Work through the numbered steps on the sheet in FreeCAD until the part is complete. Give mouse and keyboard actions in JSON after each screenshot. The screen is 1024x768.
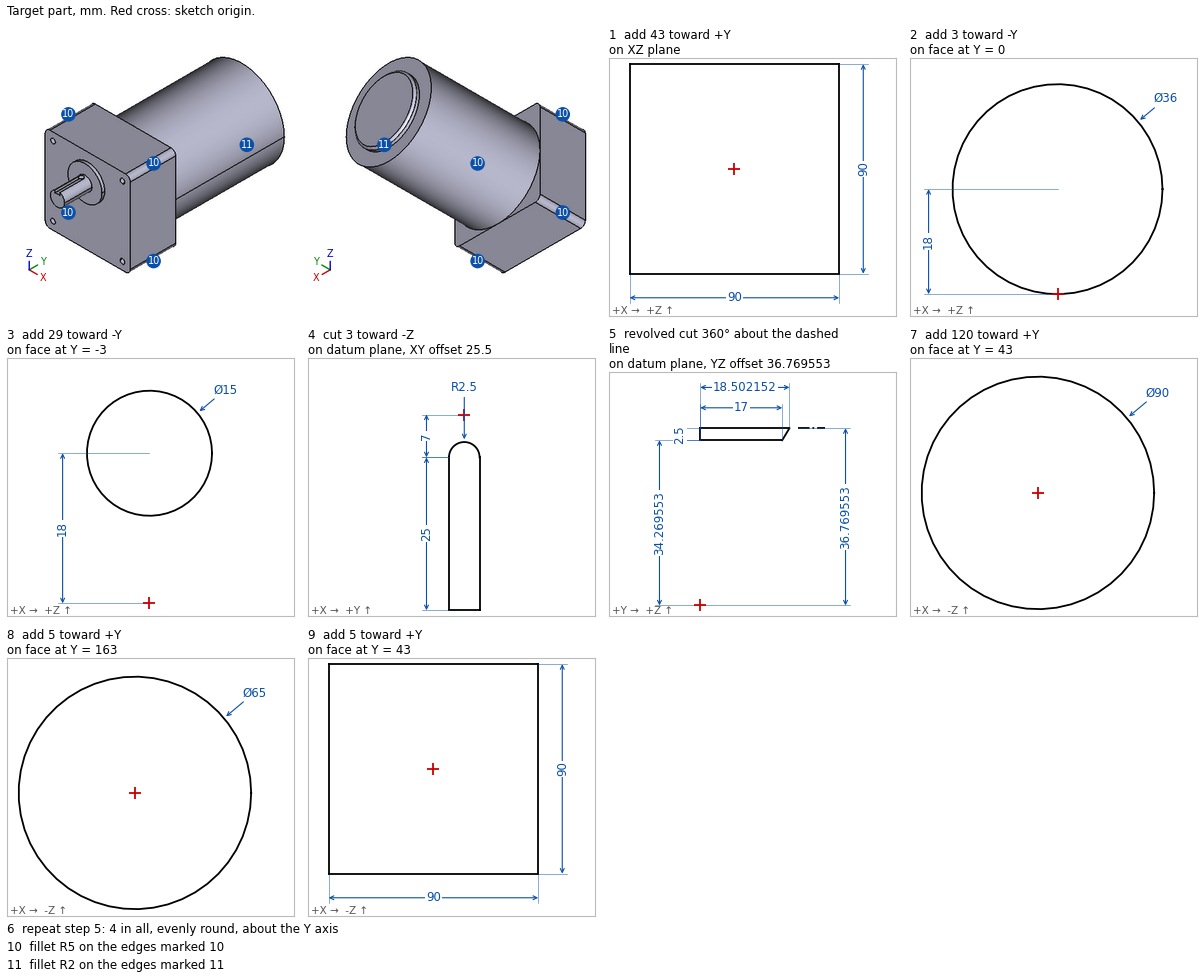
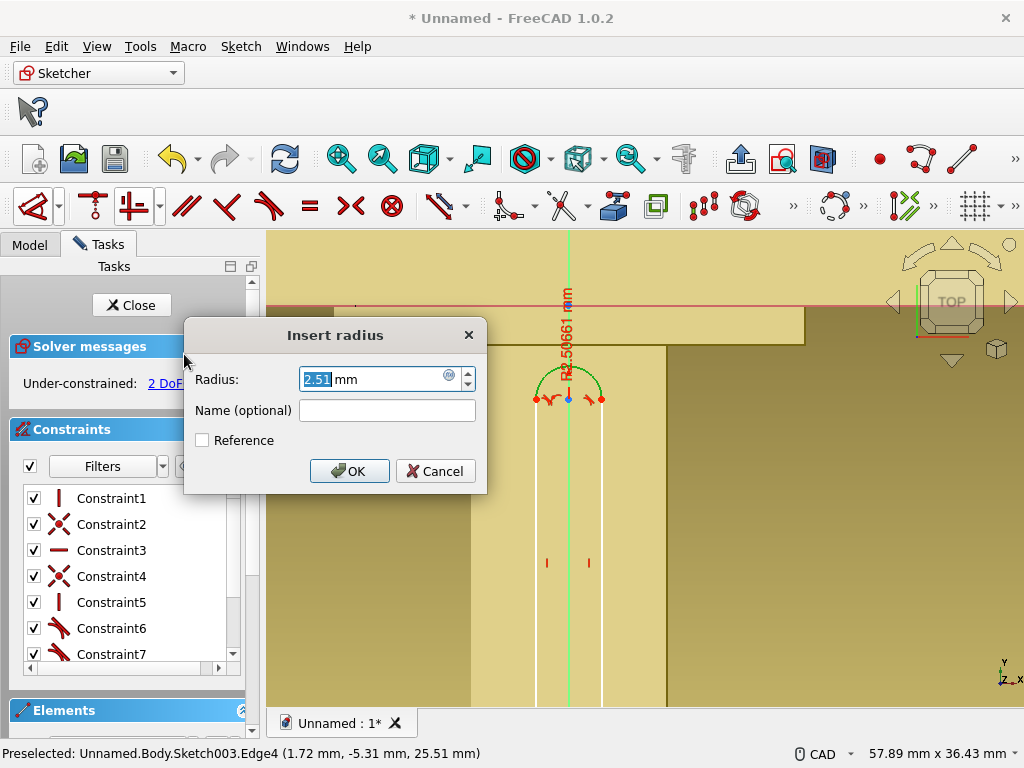
{"action": "type", "text": "2.5"}
{"action": "key", "text": "Return"}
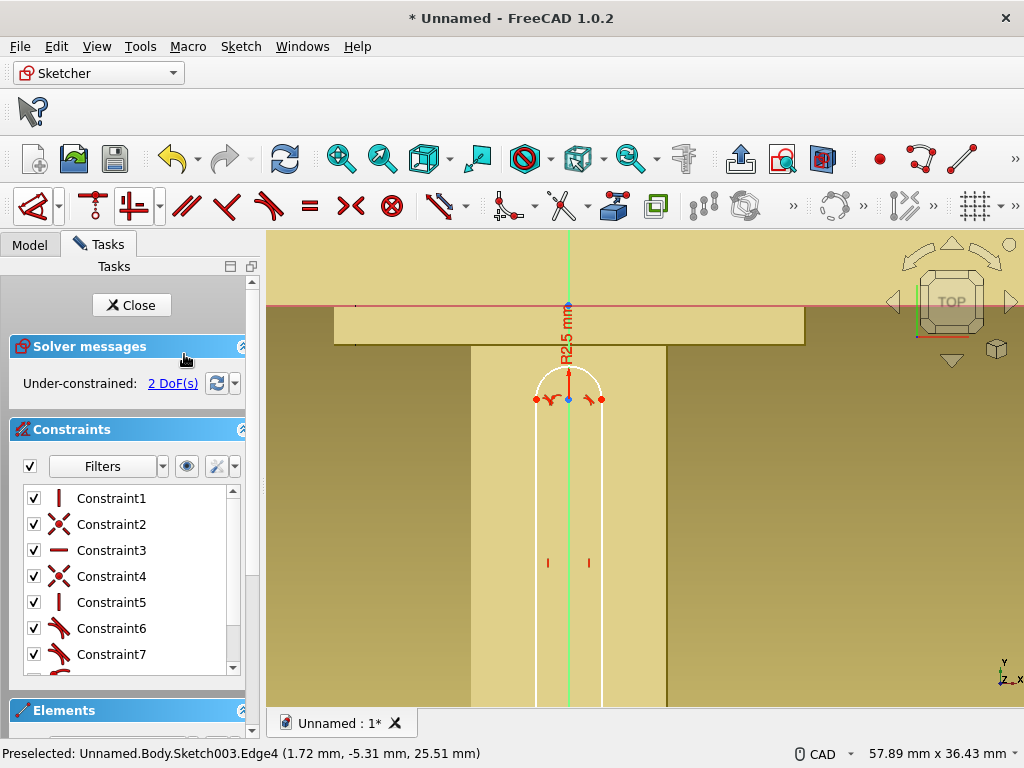
{"action": "left_click", "coordinate": [536, 497]}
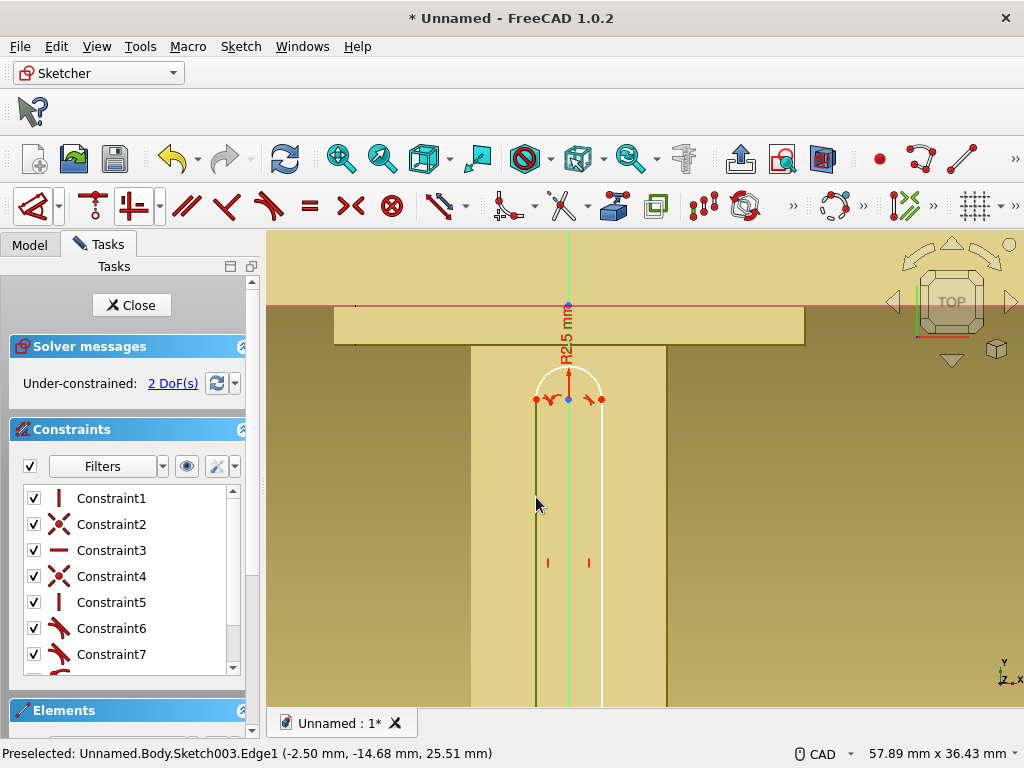
{"action": "left_click", "coordinate": [58, 206]}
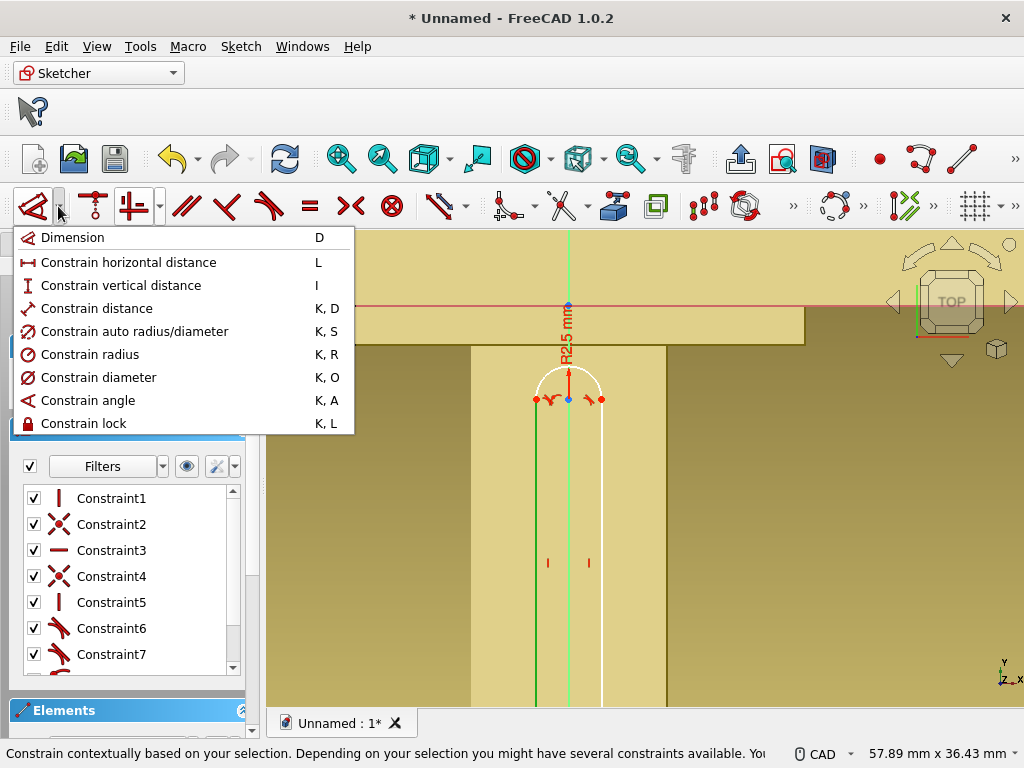
{"action": "left_click", "coordinate": [184, 286]}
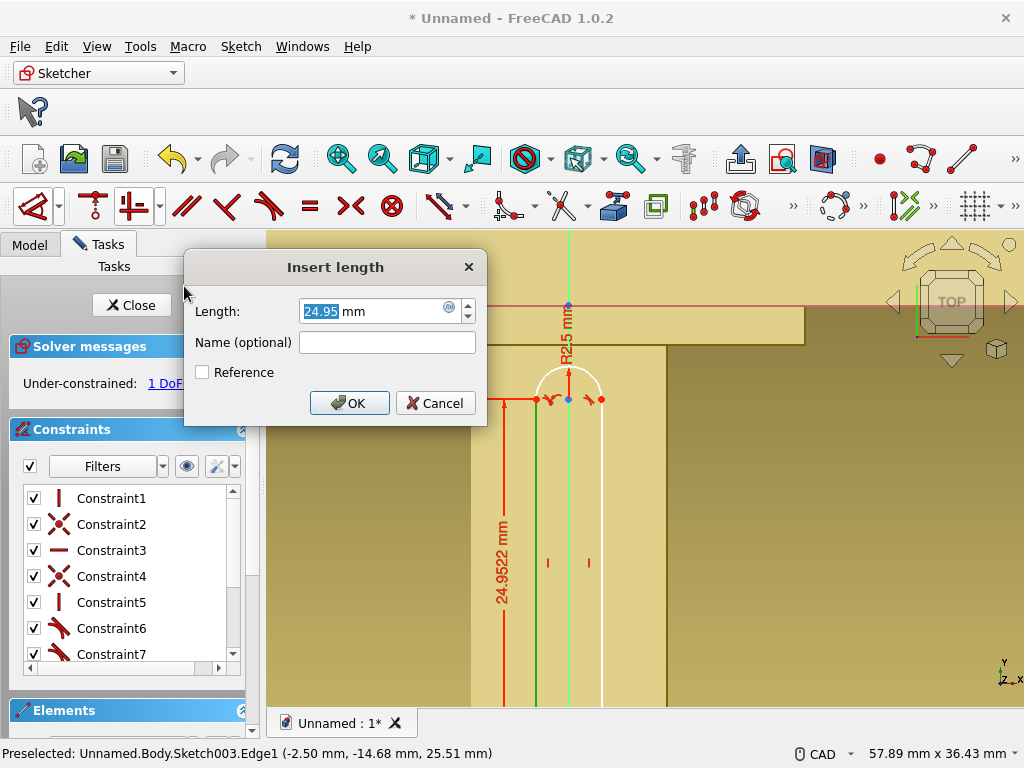
{"action": "type", "text": "25"}
{"action": "key", "text": "Return"}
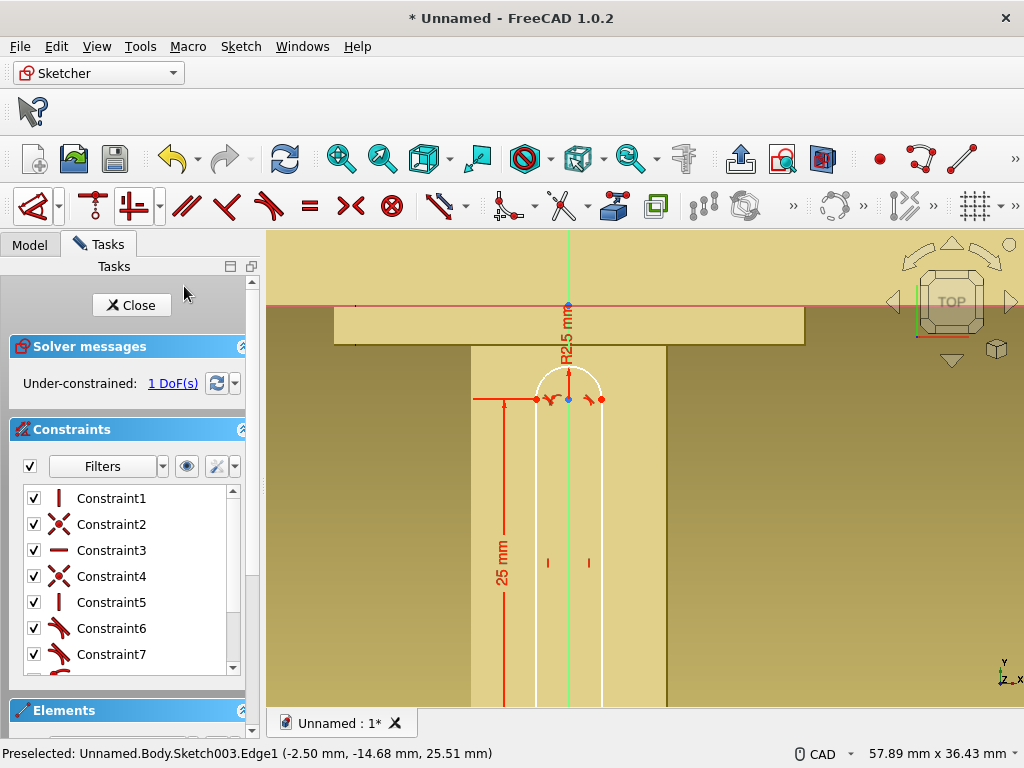
{"action": "left_click", "coordinate": [536, 399]}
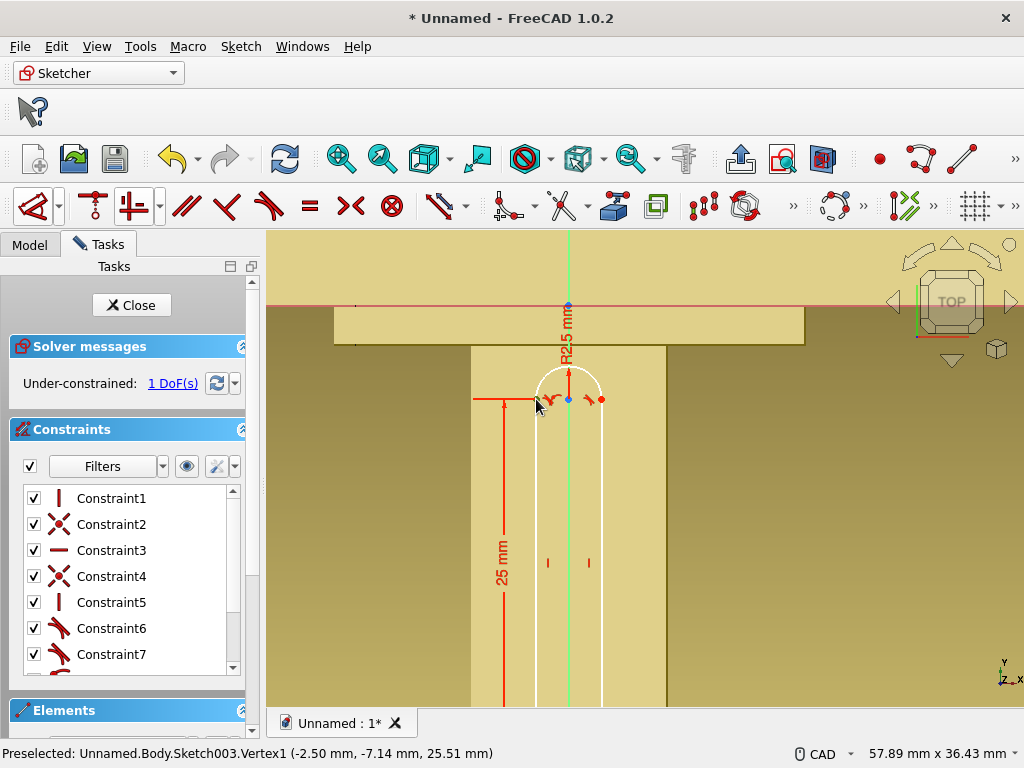
{"action": "left_click", "coordinate": [58, 206]}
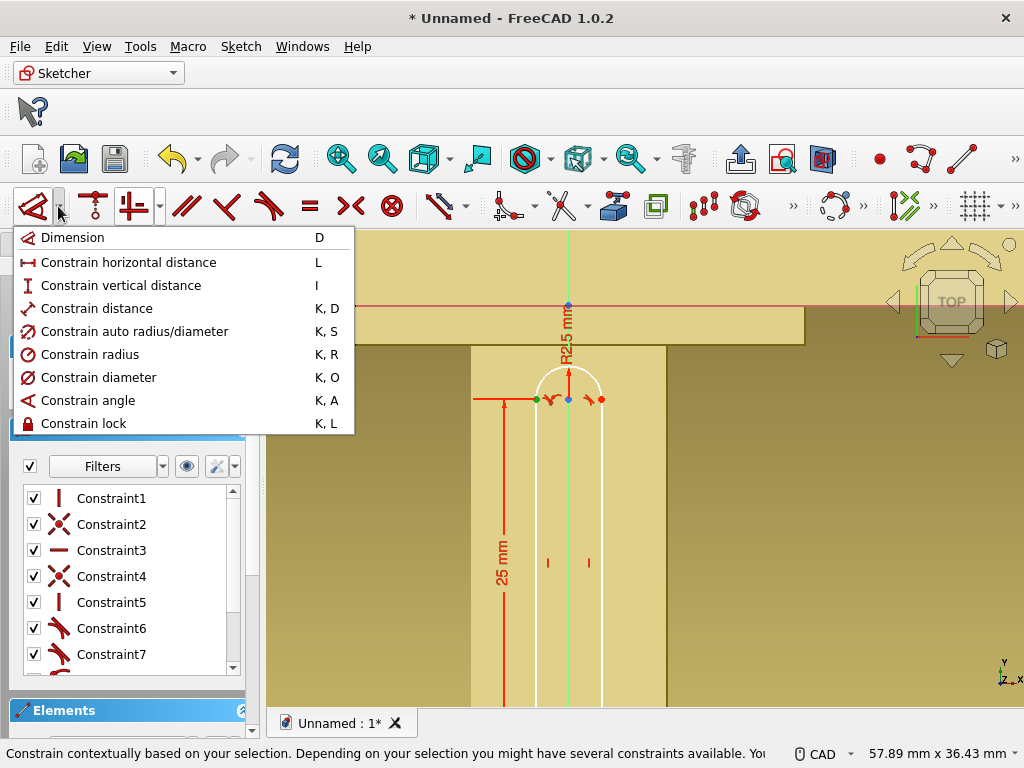
{"action": "left_click", "coordinate": [184, 286]}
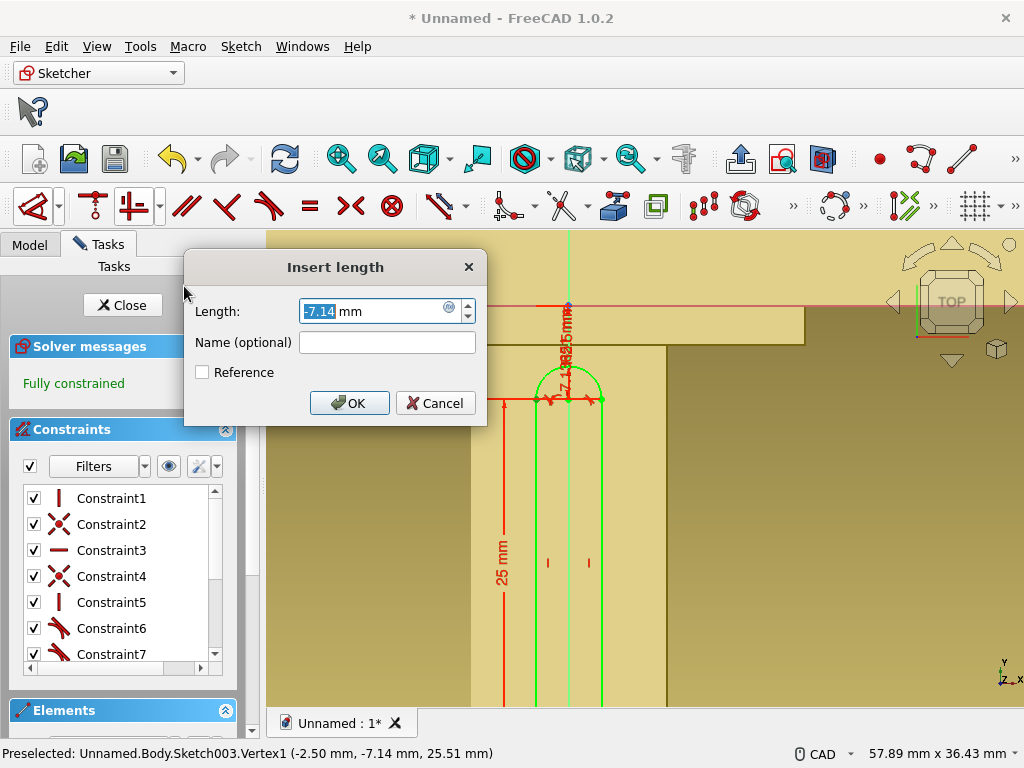
{"action": "type", "text": "-7"}
{"action": "key", "text": "Return"}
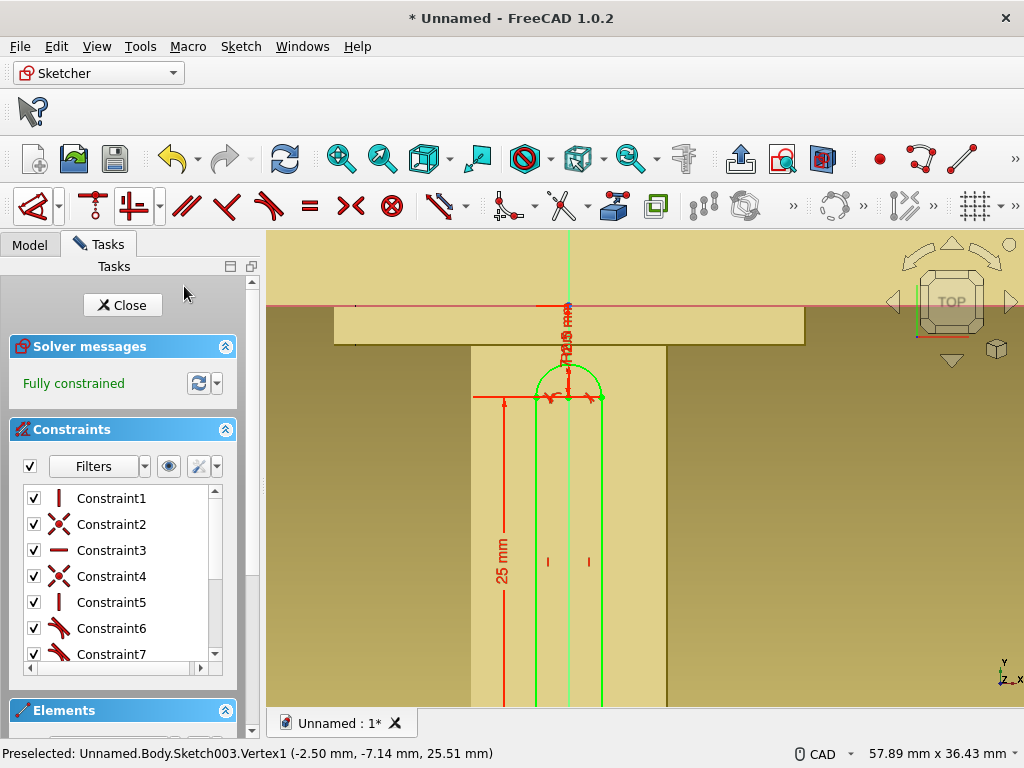
{"action": "left_click", "coordinate": [123, 305]}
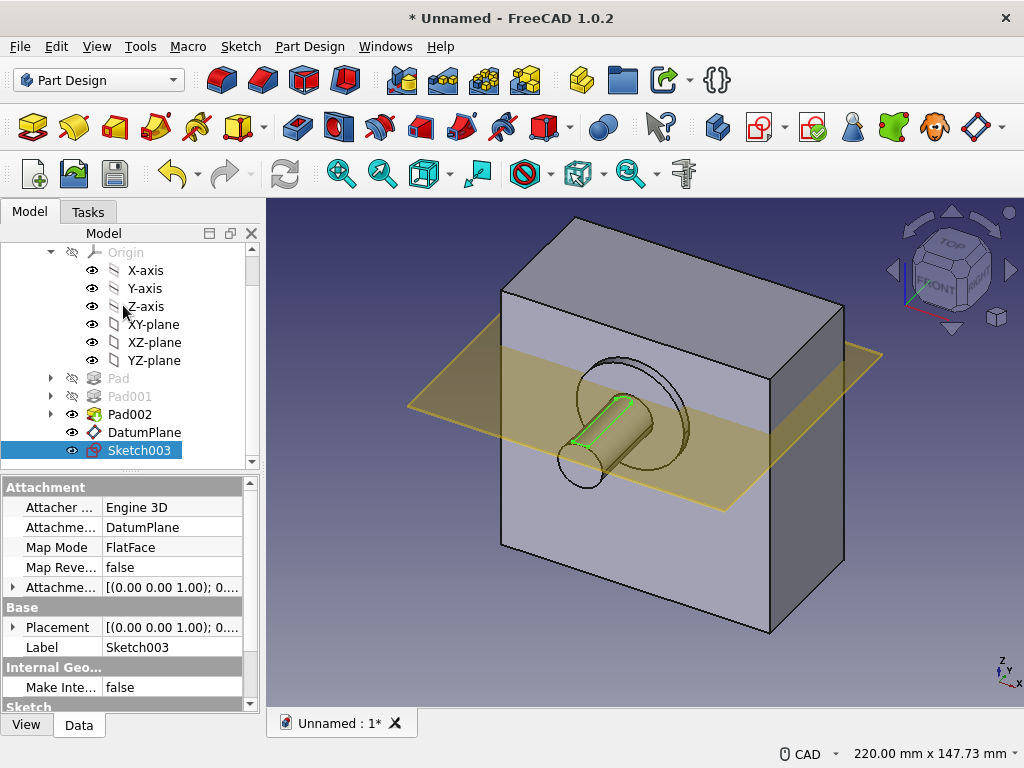
{"action": "left_click", "coordinate": [298, 128]}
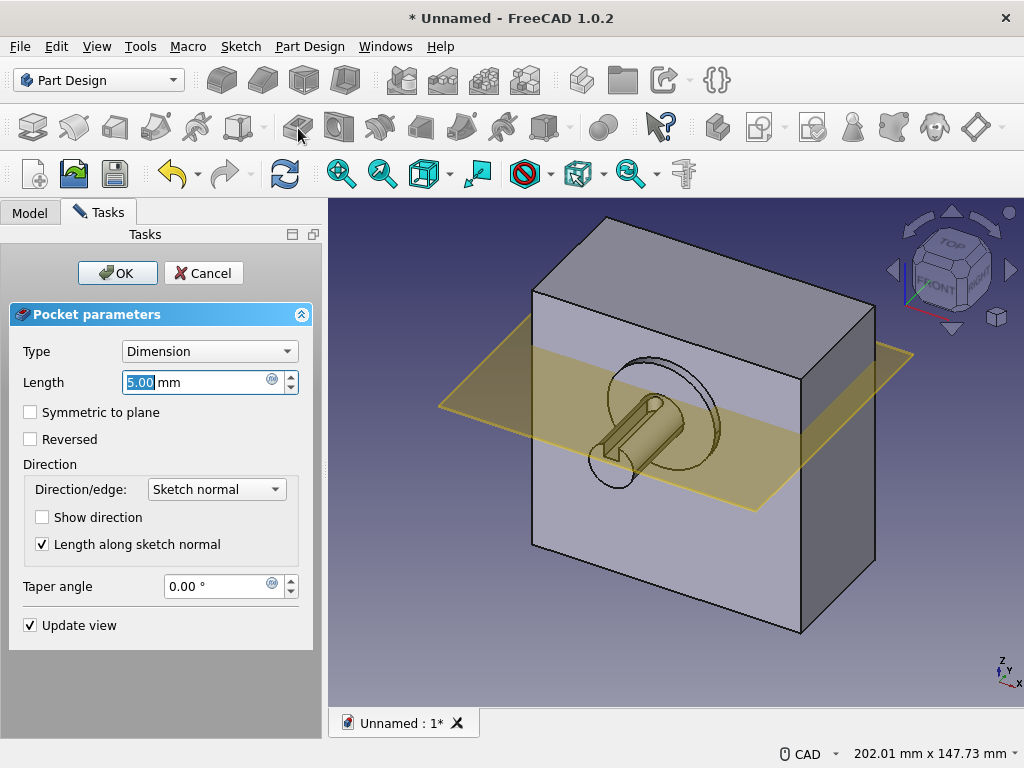
{"action": "type", "text": "3"}
{"action": "key", "text": "Tab"}